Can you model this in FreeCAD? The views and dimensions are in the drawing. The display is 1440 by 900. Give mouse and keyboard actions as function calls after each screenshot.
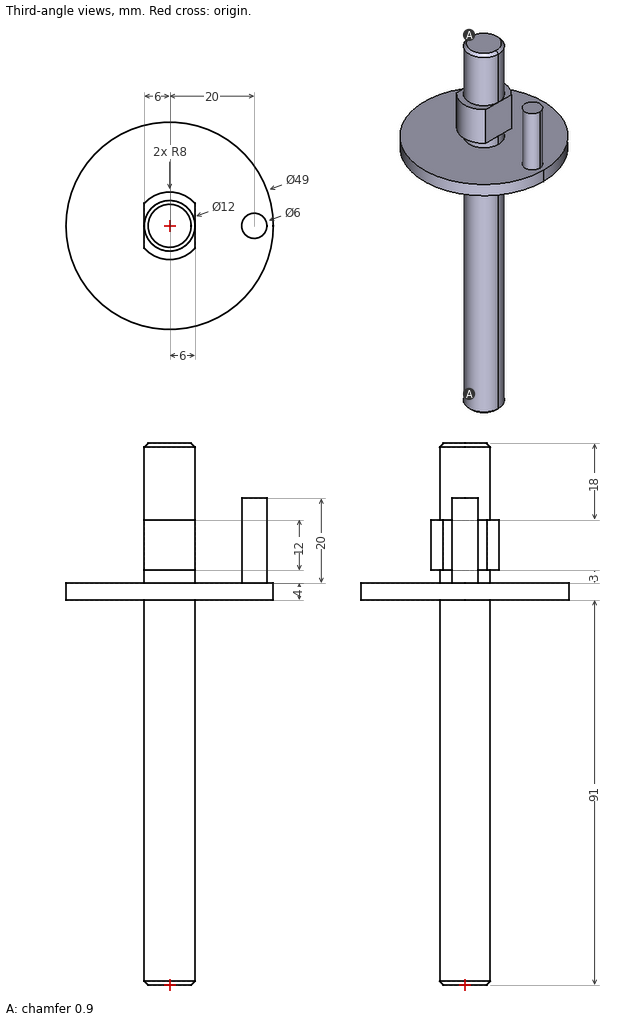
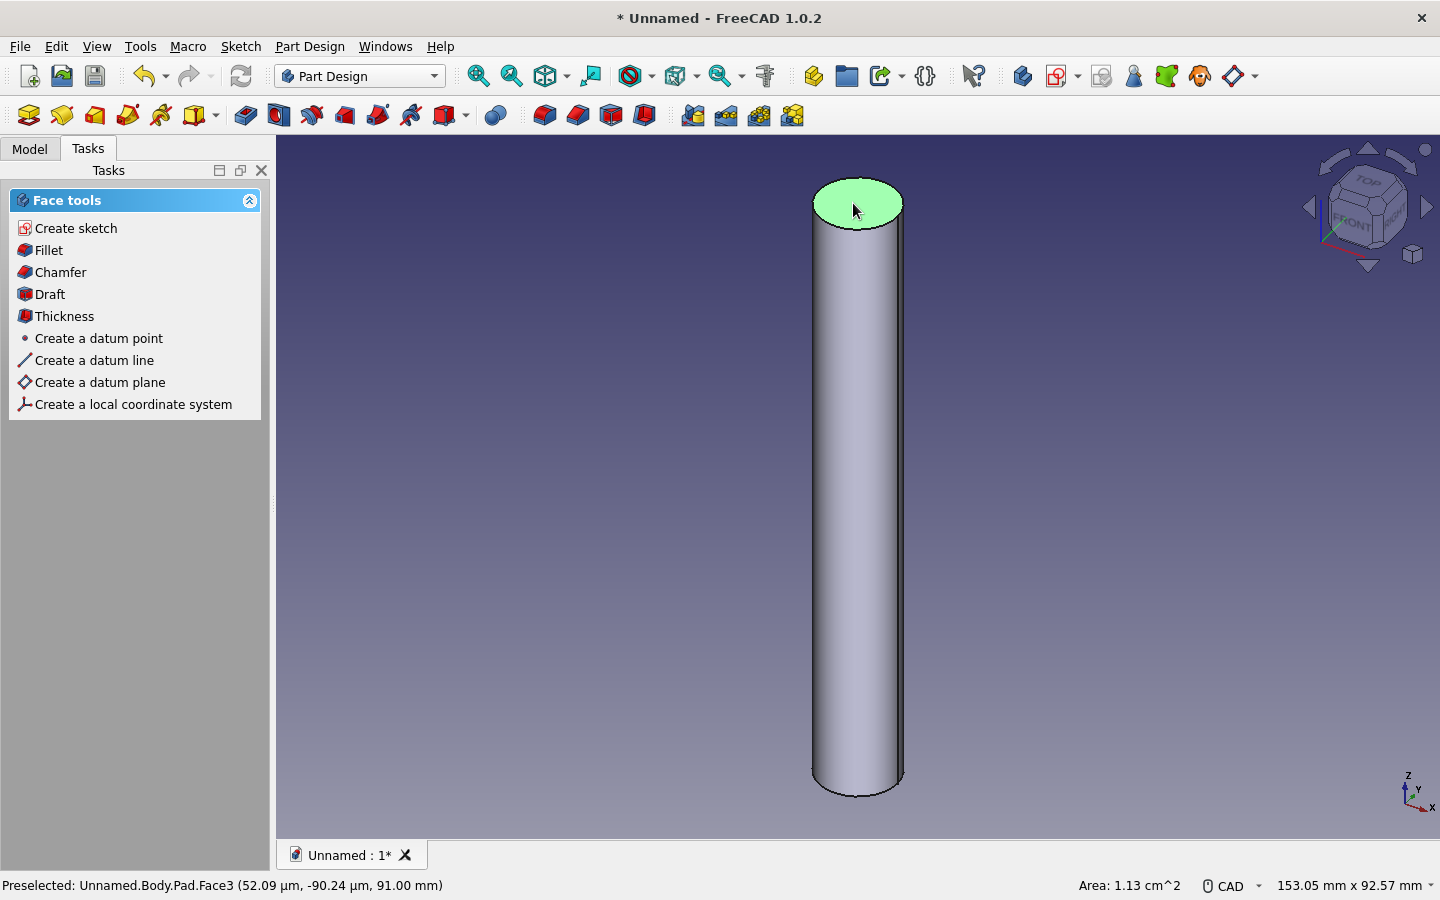
click(1056, 76)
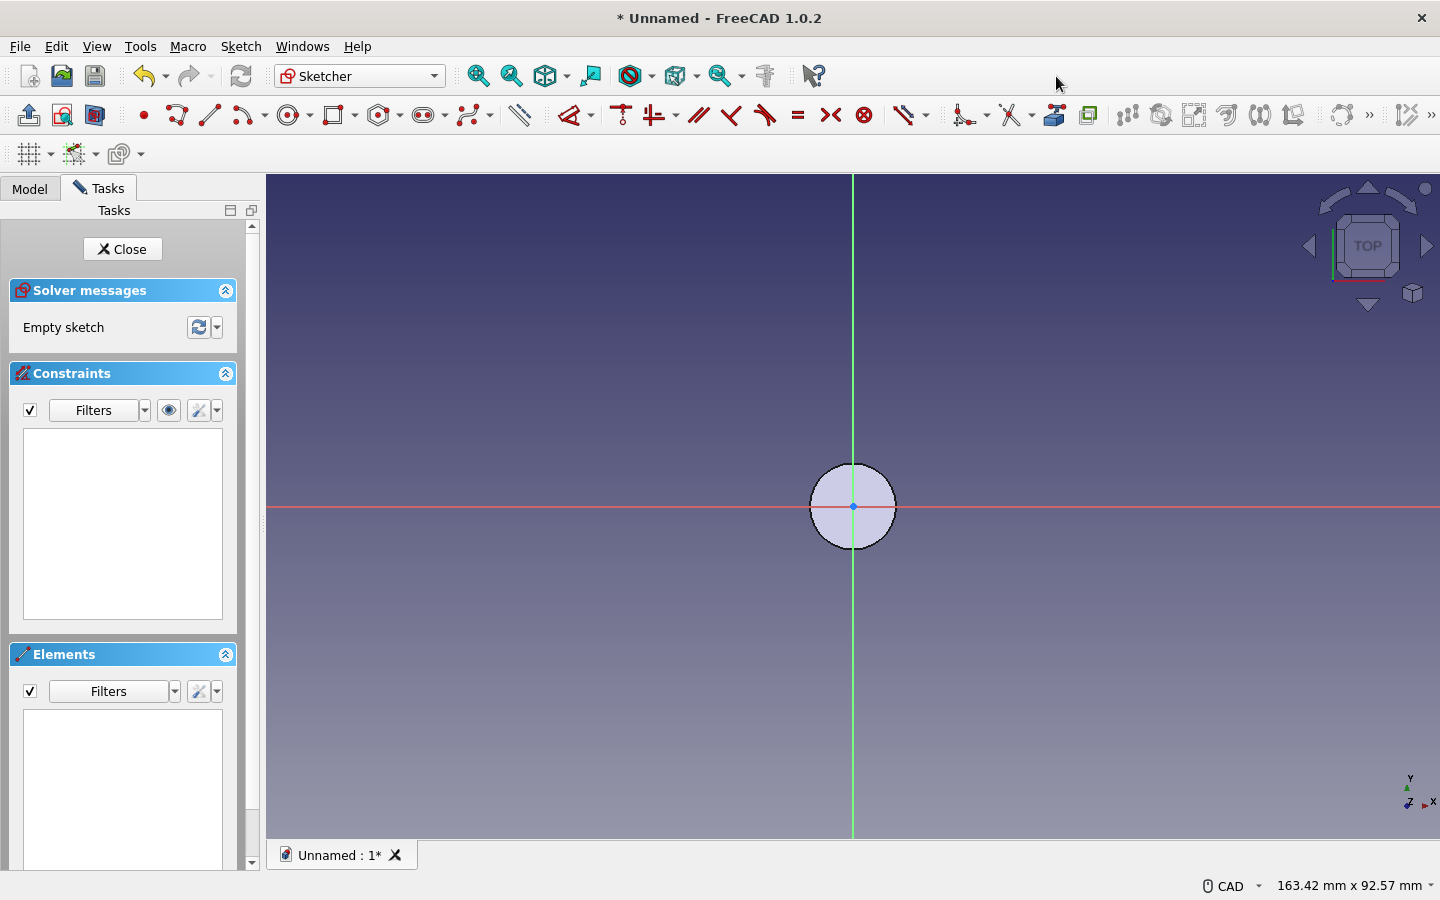
click(288, 116)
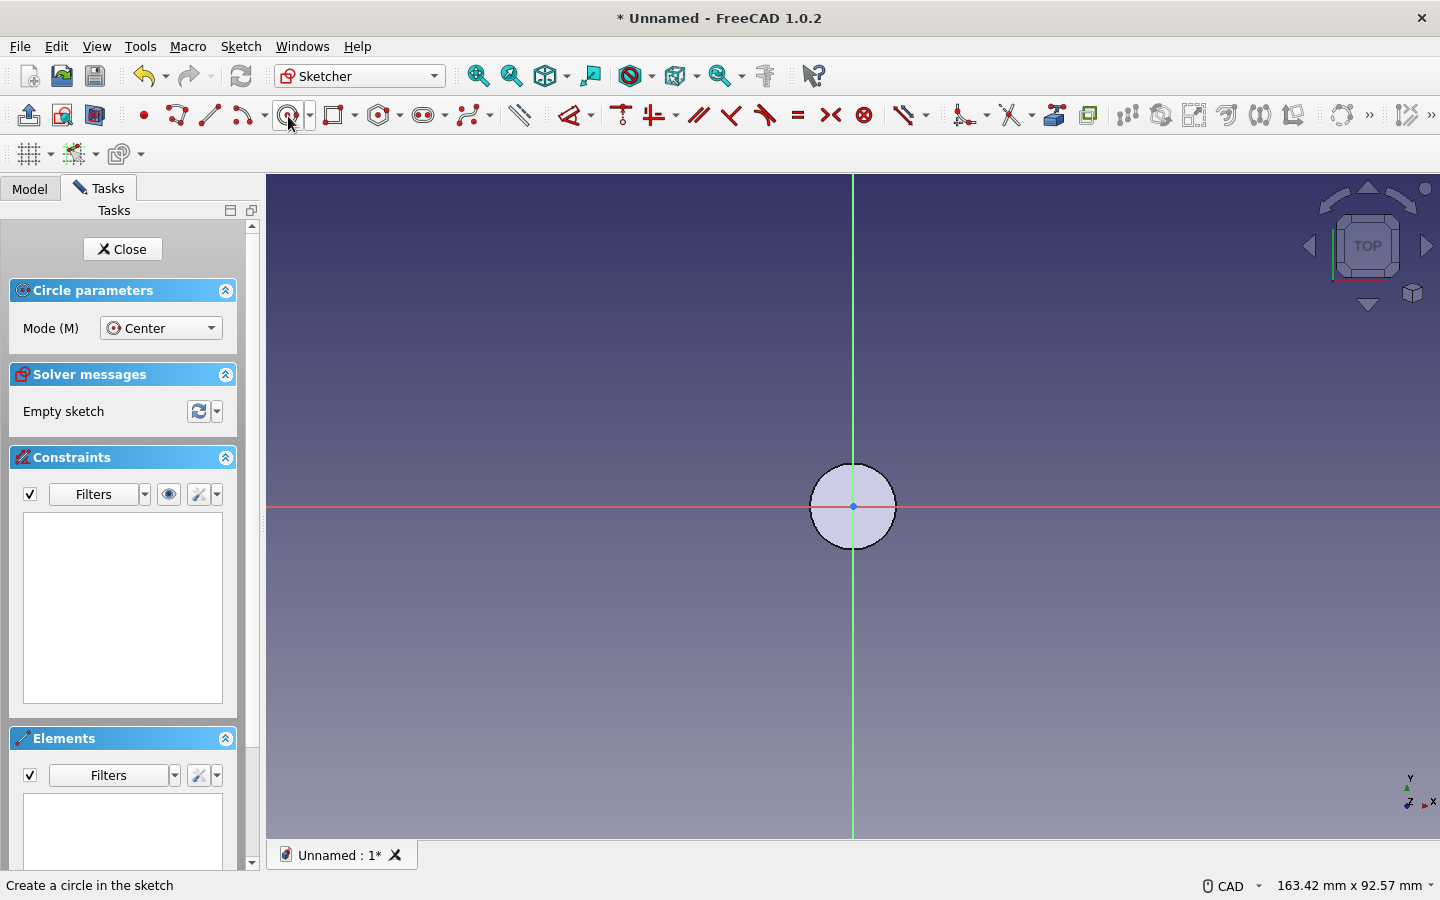
click(853, 506)
click(977, 382)
key(Escape)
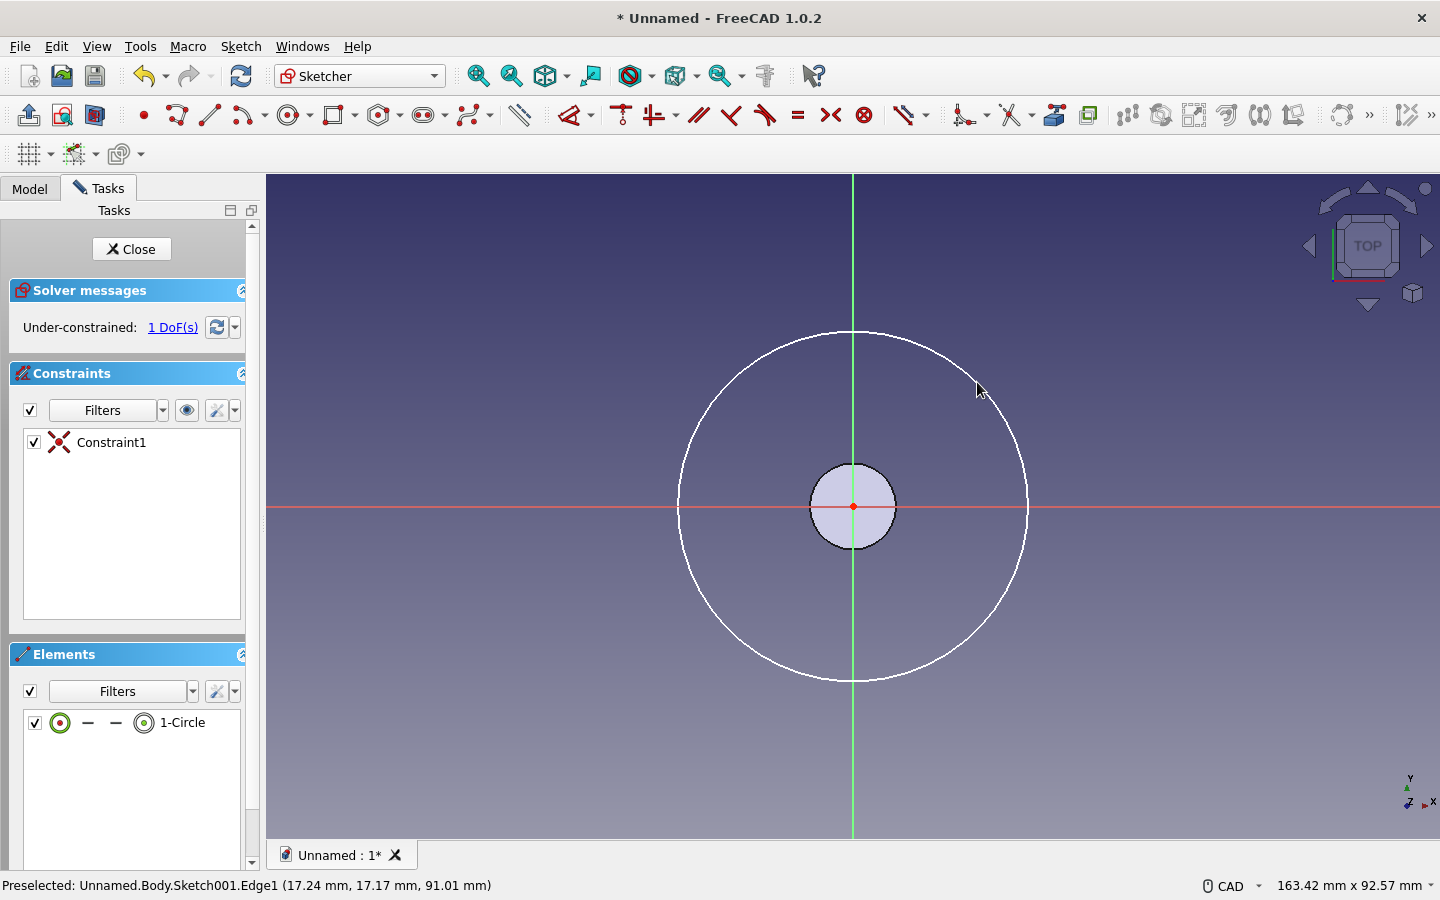
click(976, 382)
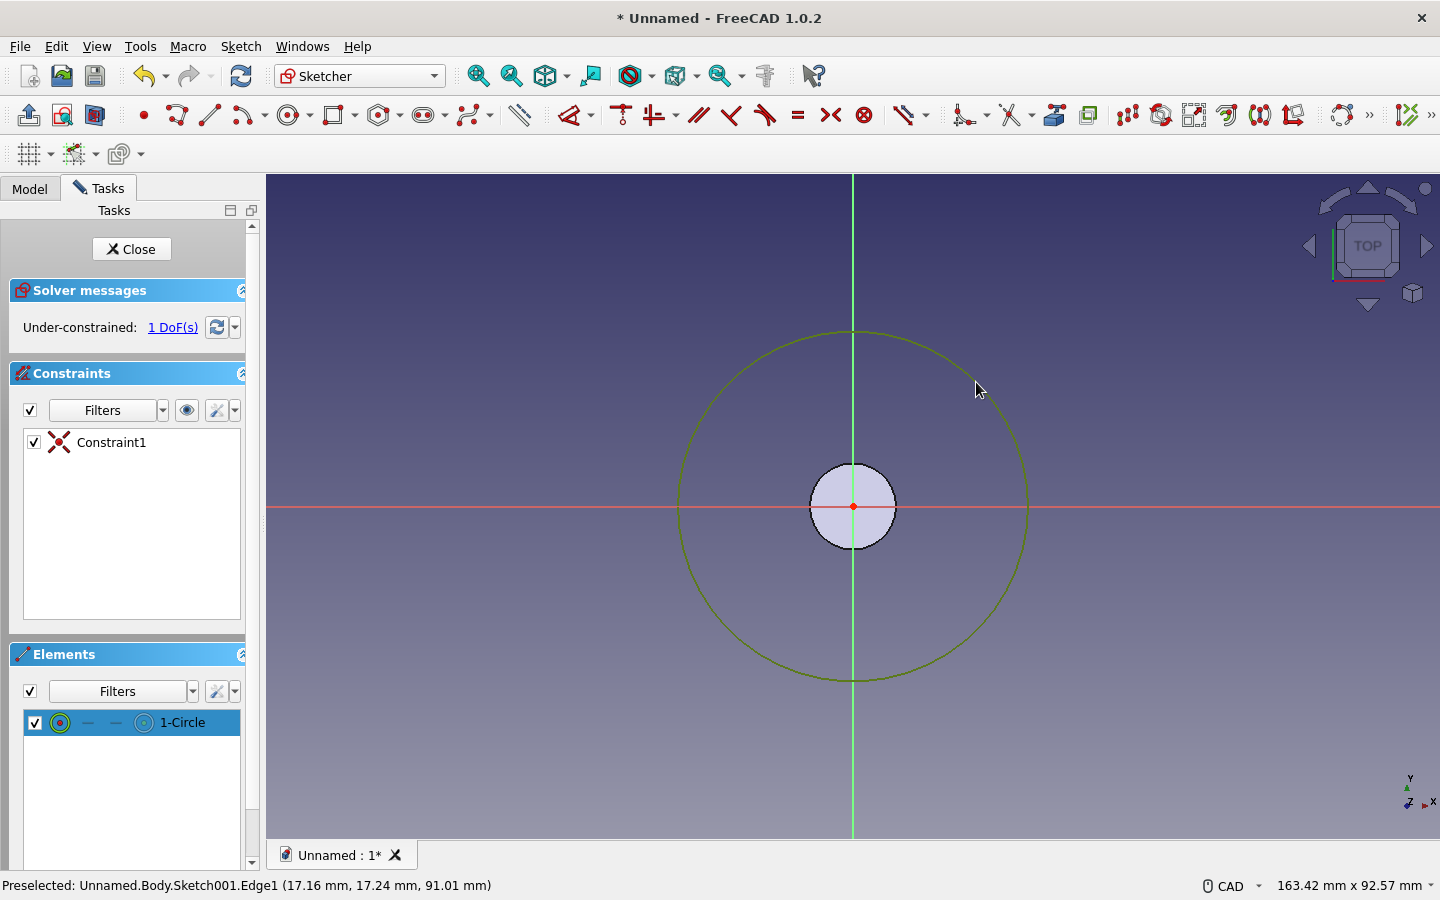
click(590, 116)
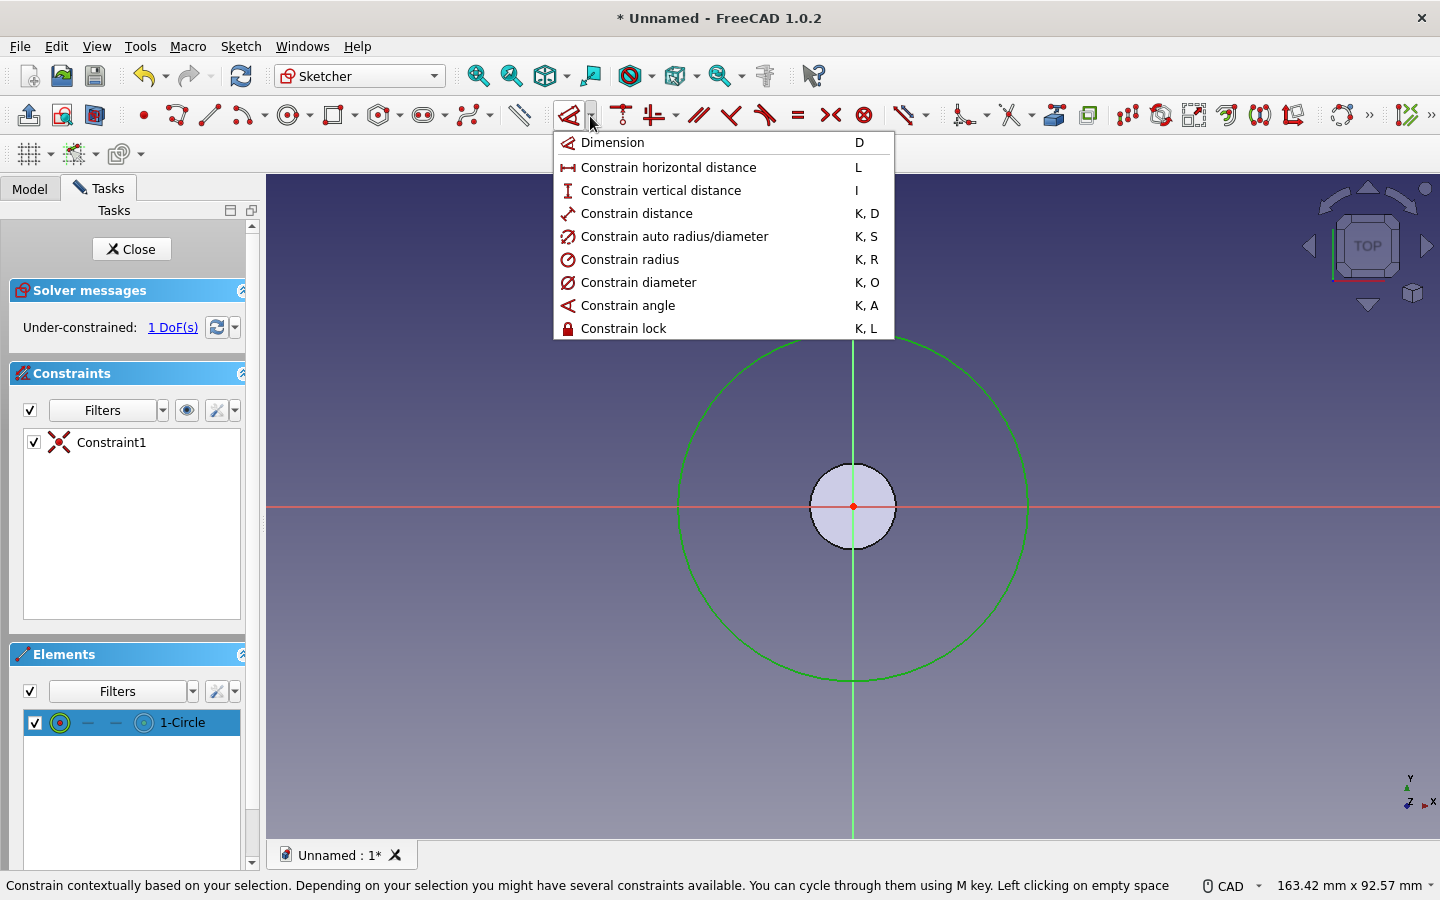
click(724, 282)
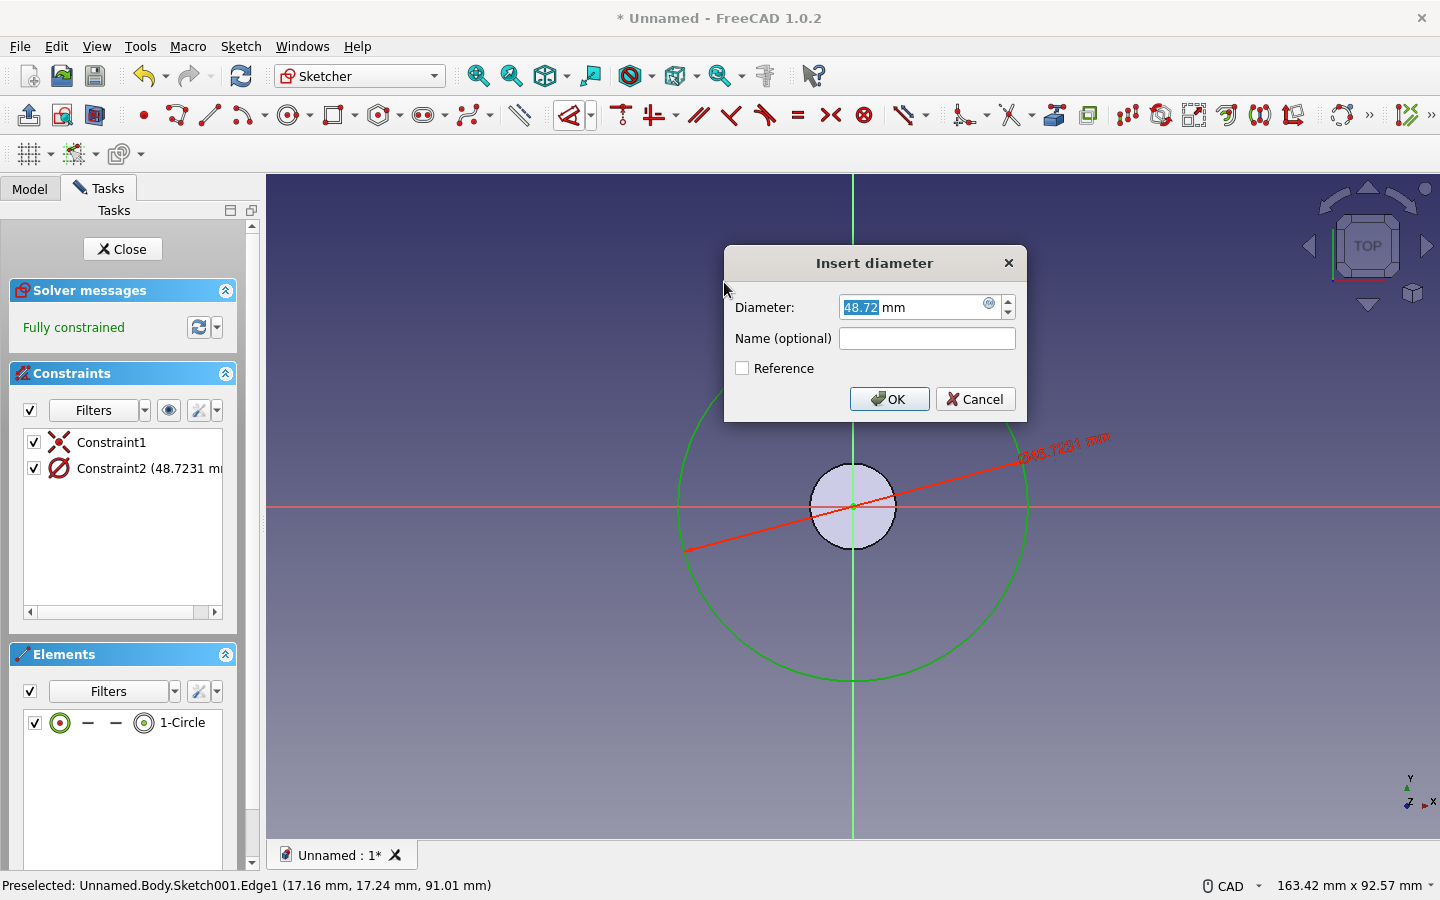
text(49)
key(Return)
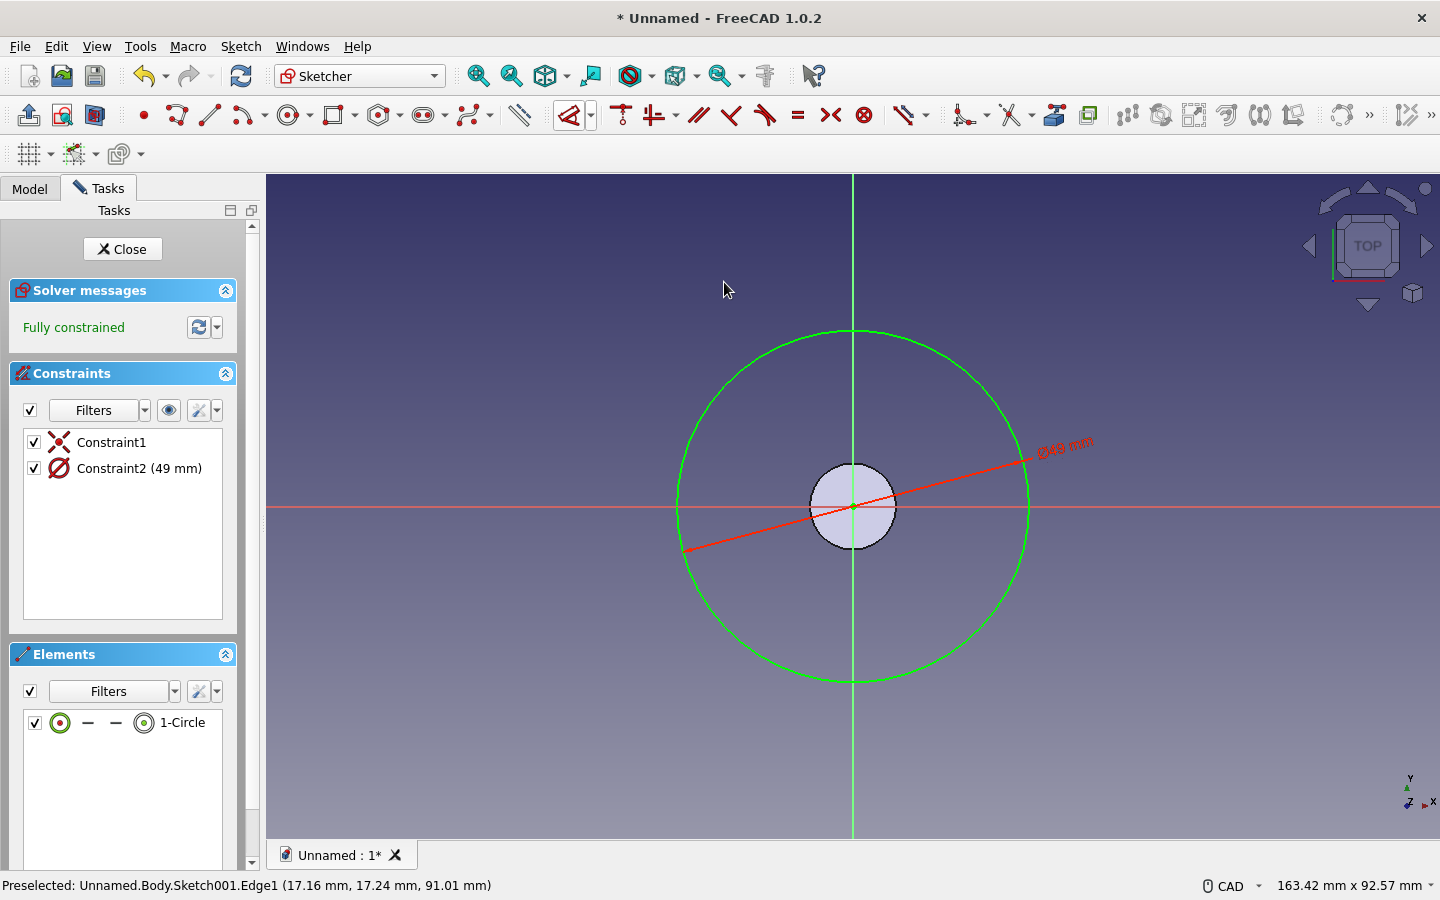
click(123, 249)